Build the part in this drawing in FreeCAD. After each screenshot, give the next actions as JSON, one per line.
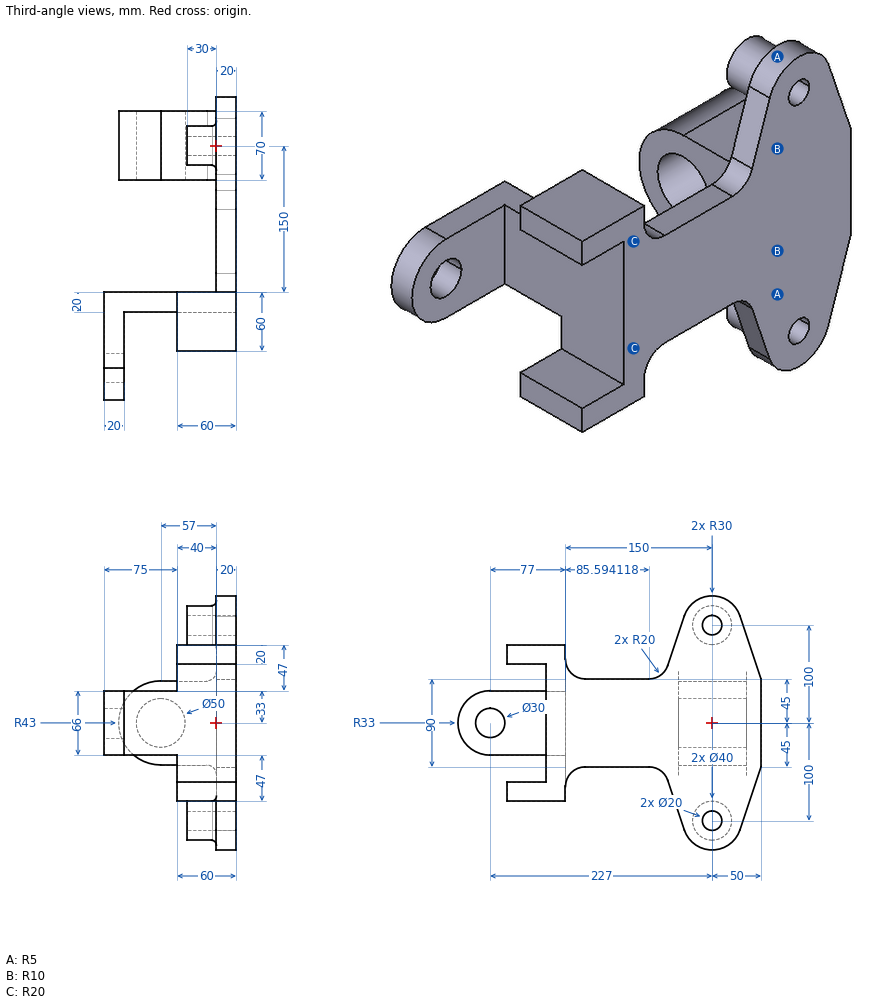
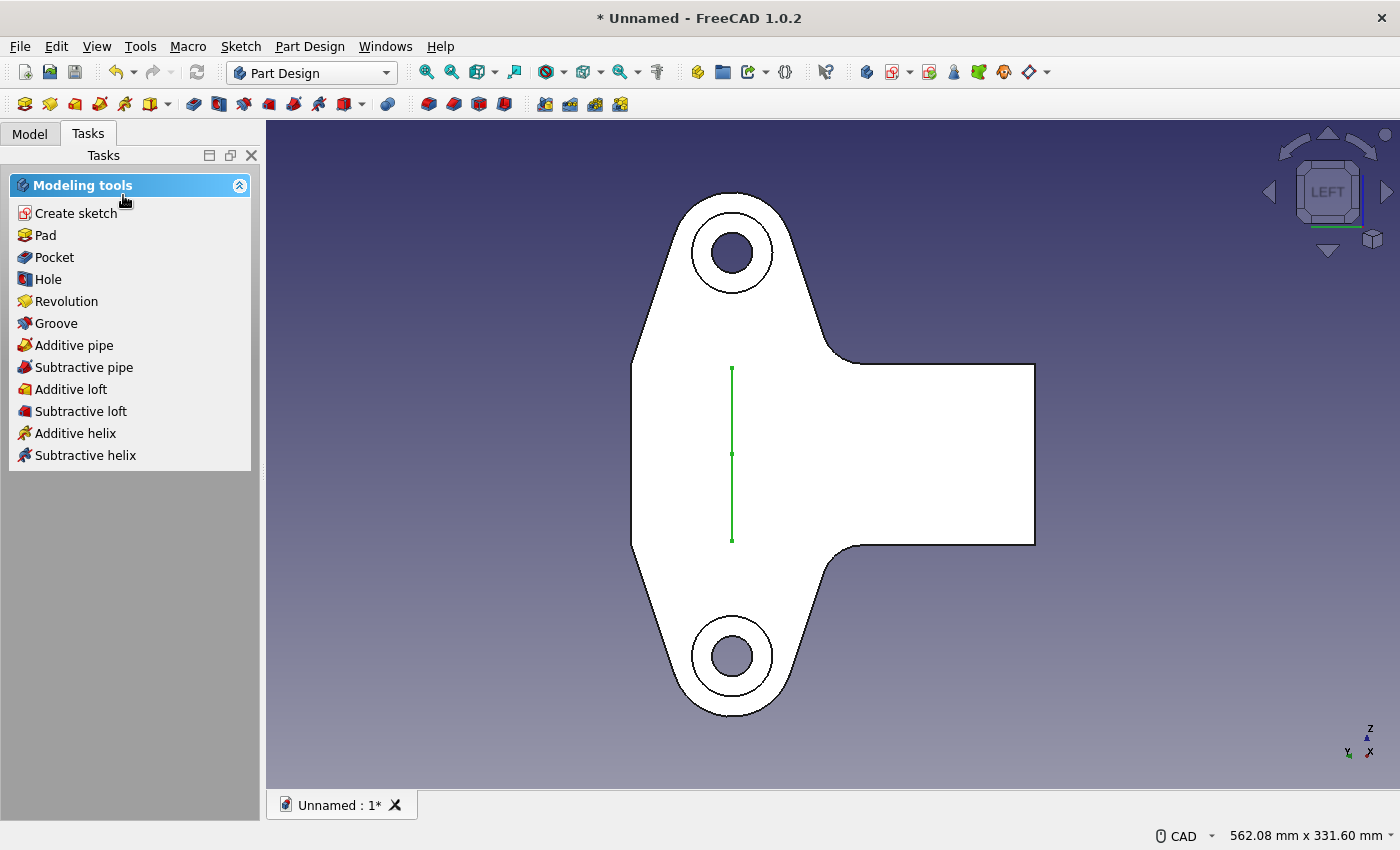
{"action": "left_click", "coordinate": [25, 104]}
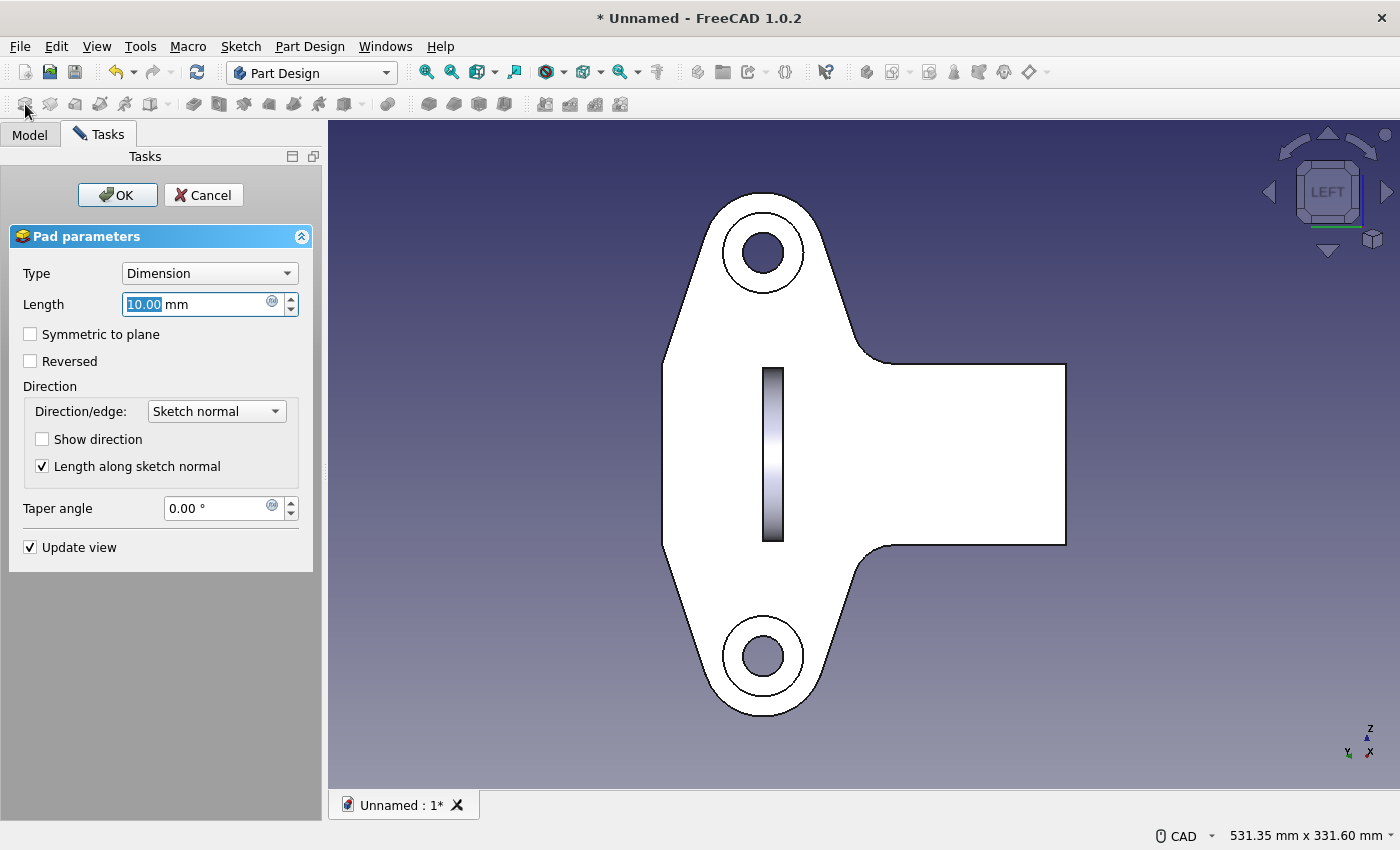
{"action": "type", "text": "70"}
{"action": "key", "text": "Tab"}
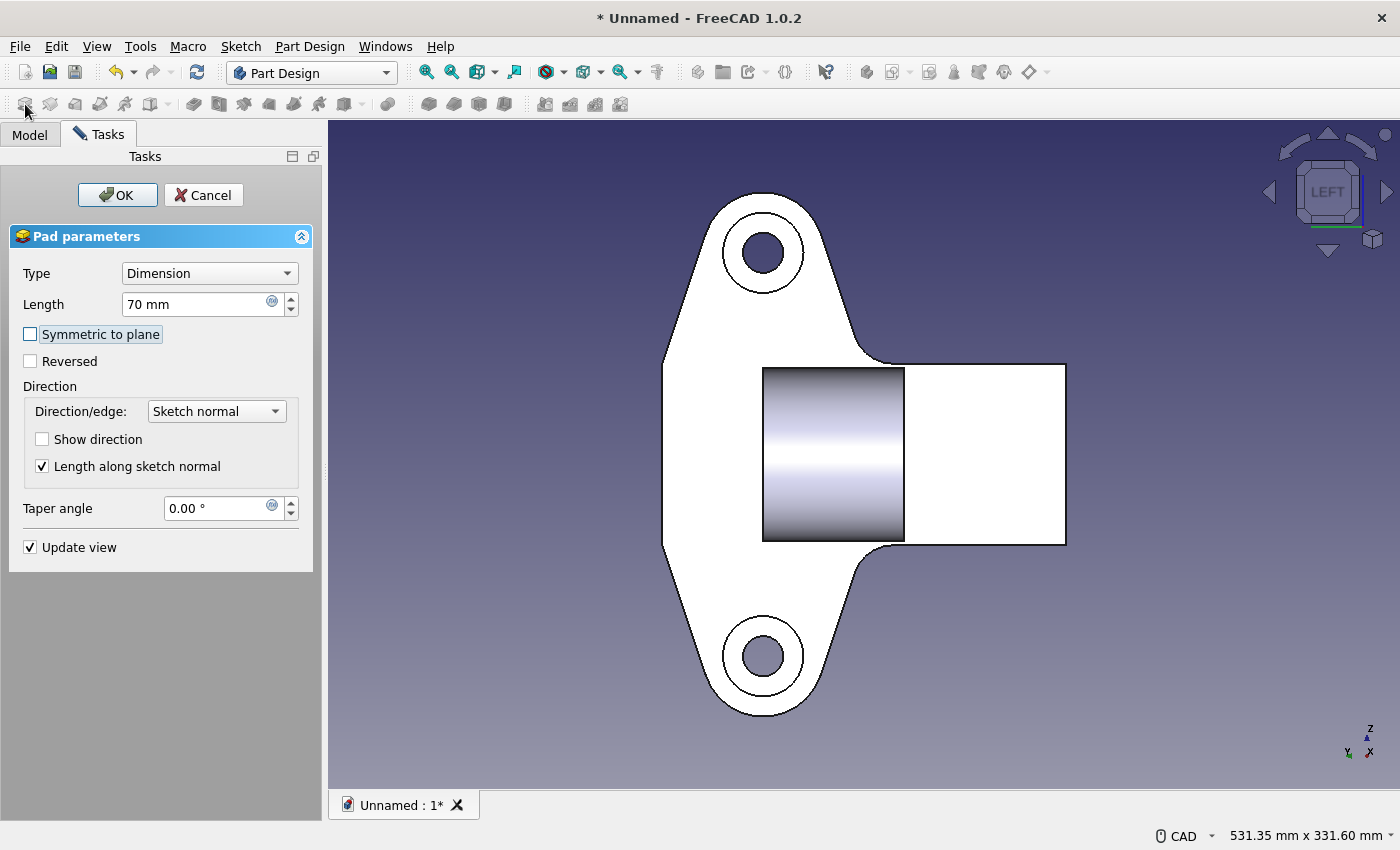
{"action": "left_click", "coordinate": [31, 334]}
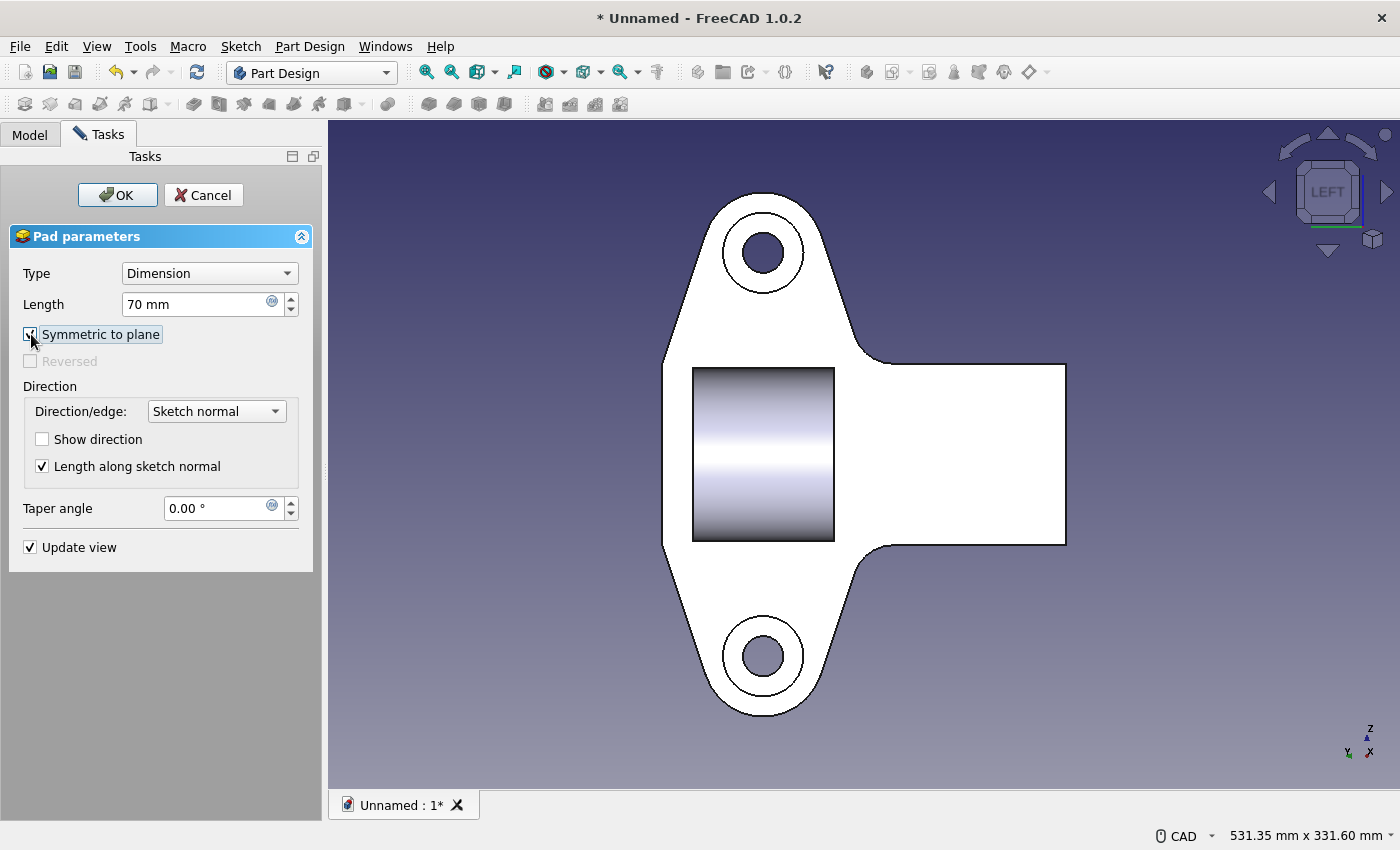
{"action": "left_click", "coordinate": [118, 195]}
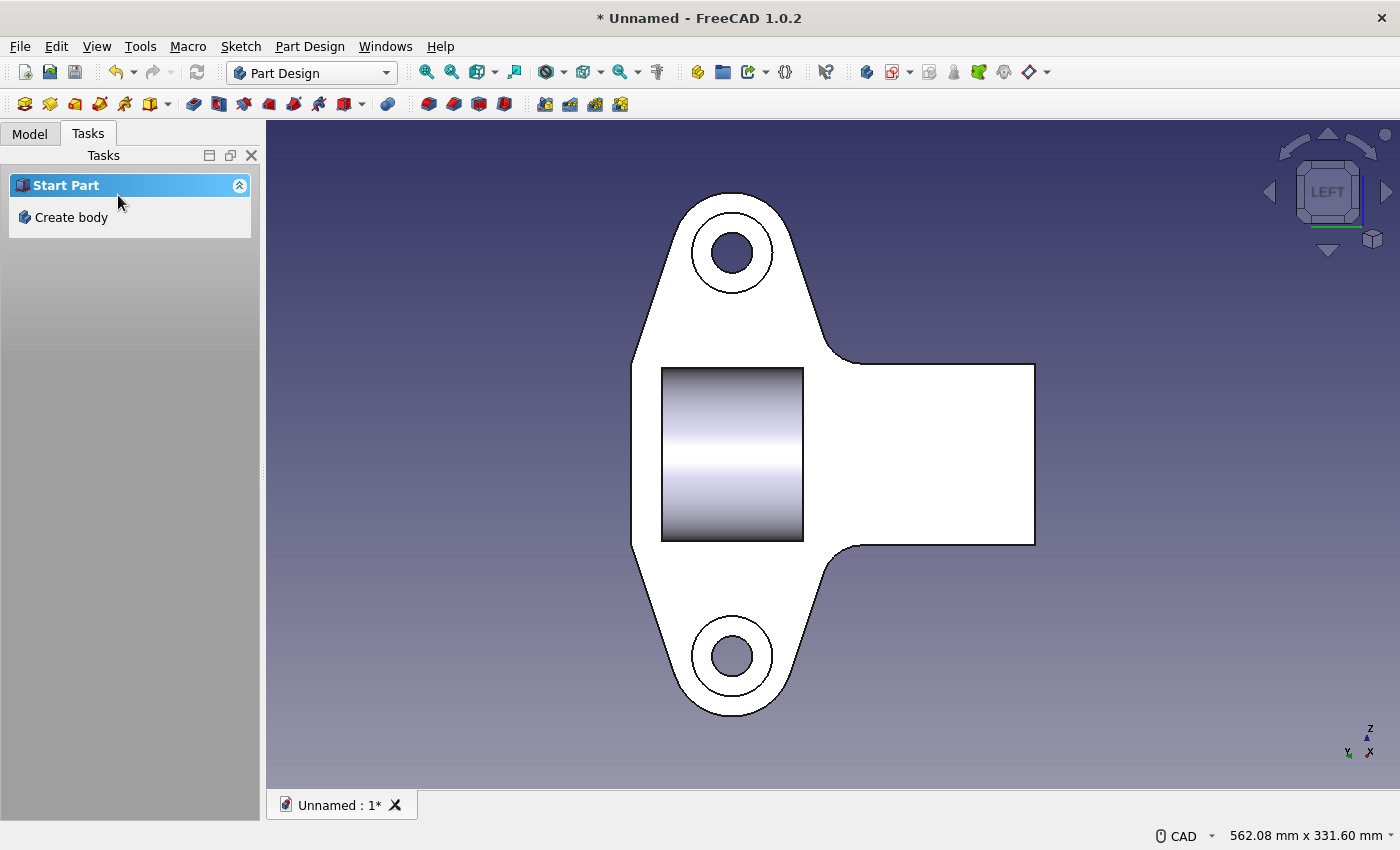
{"action": "key", "text": "0"}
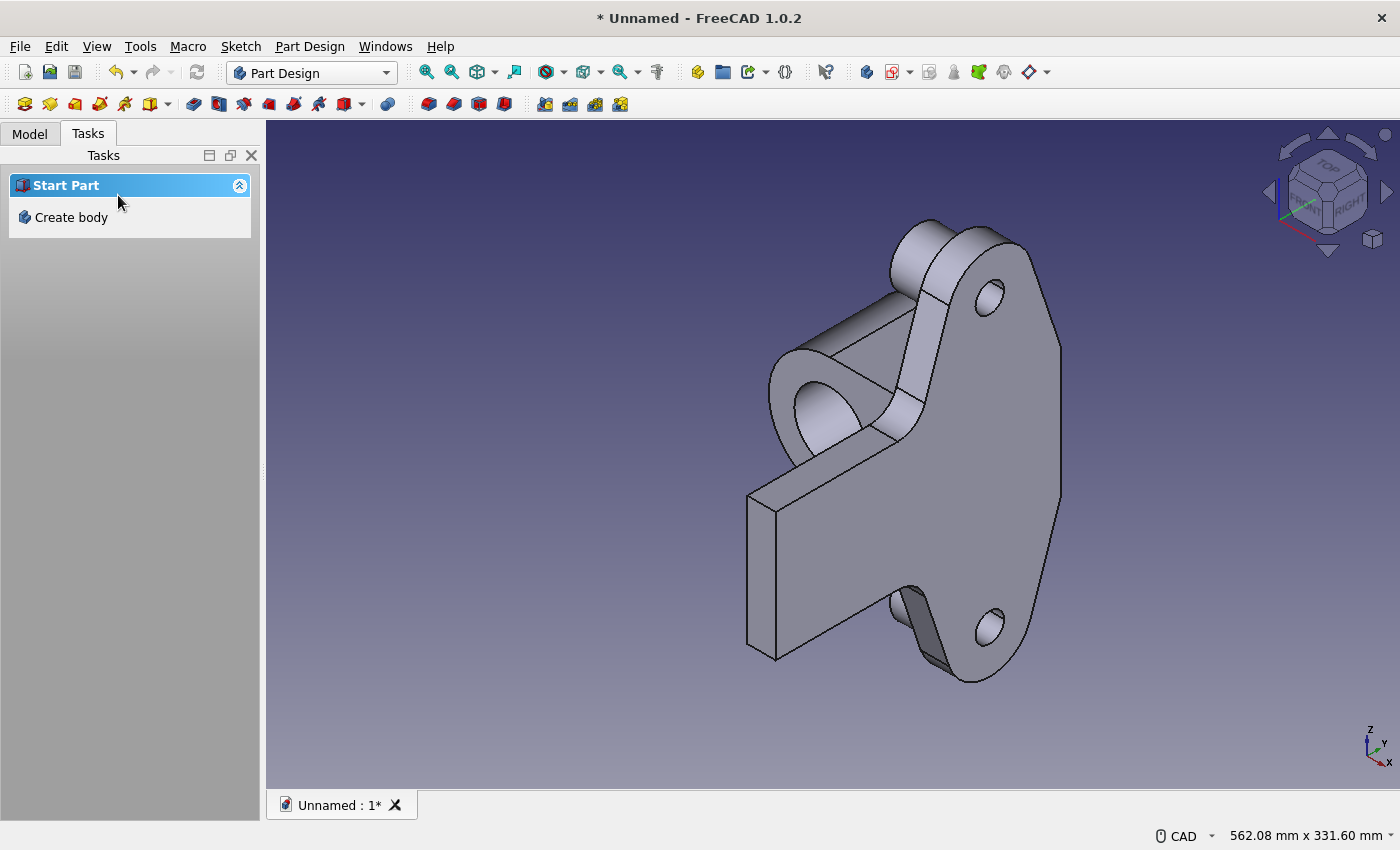
{"action": "left_click", "coordinate": [427, 72]}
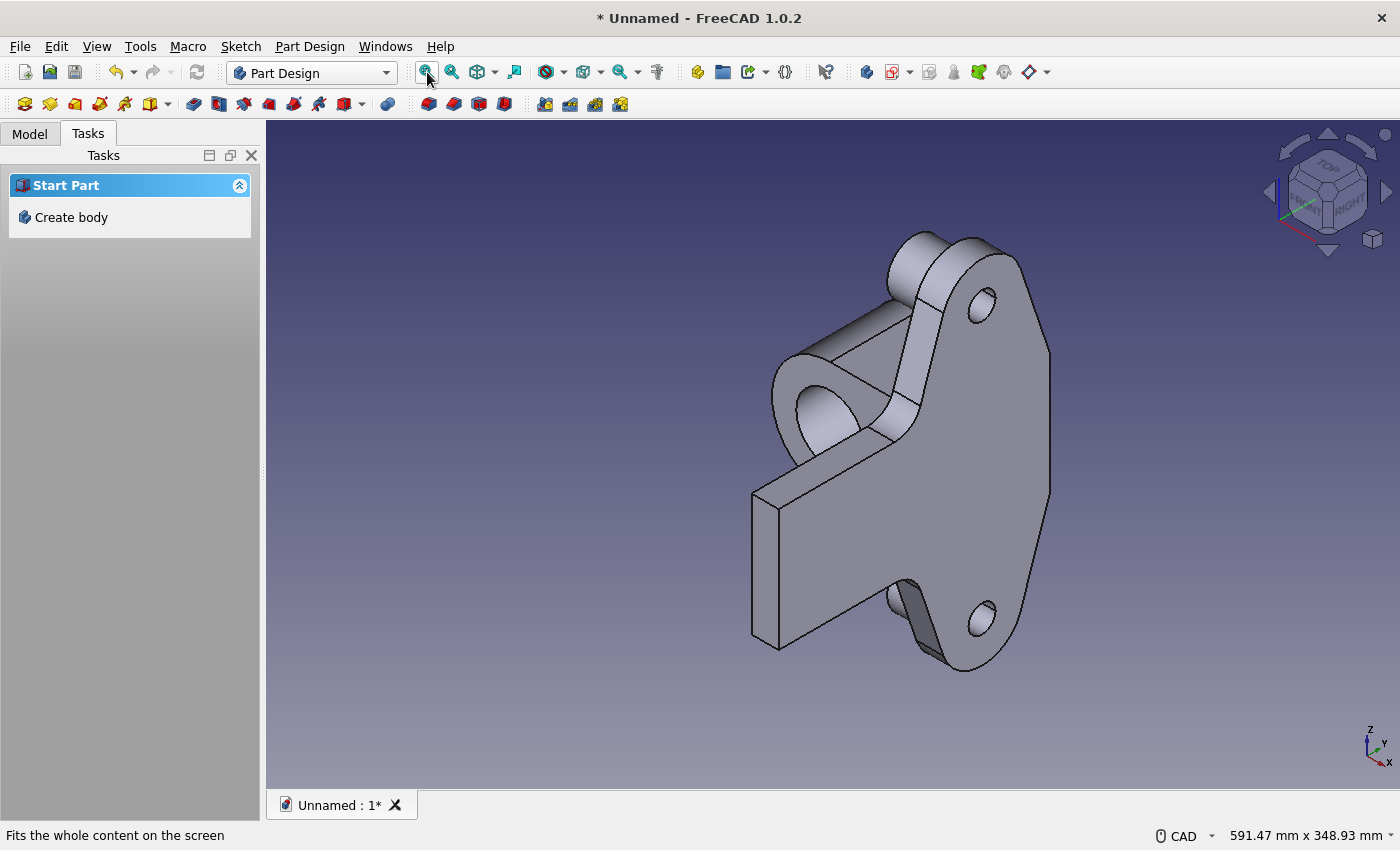
{"action": "left_click", "coordinate": [765, 611]}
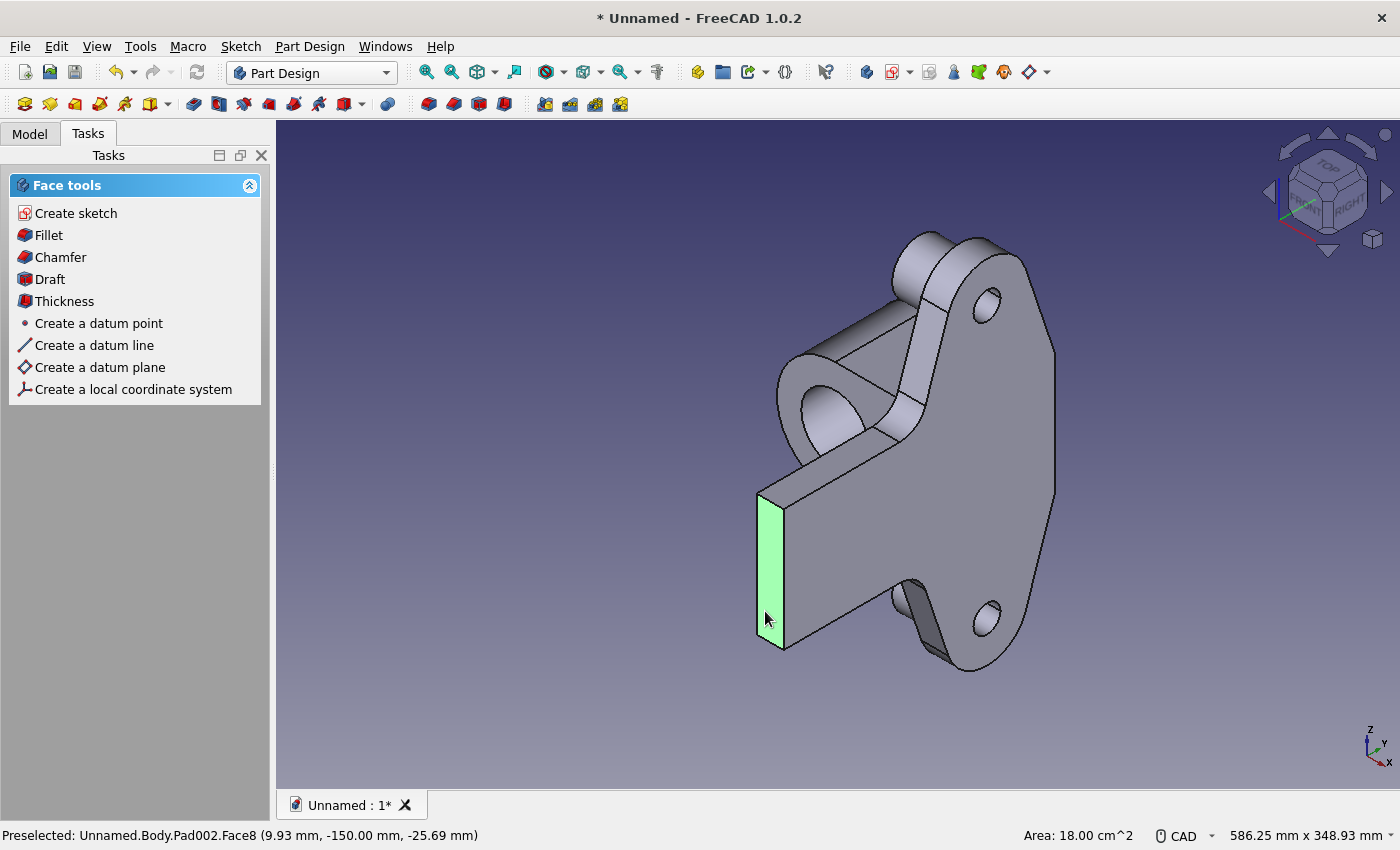
{"action": "left_click", "coordinate": [892, 72]}